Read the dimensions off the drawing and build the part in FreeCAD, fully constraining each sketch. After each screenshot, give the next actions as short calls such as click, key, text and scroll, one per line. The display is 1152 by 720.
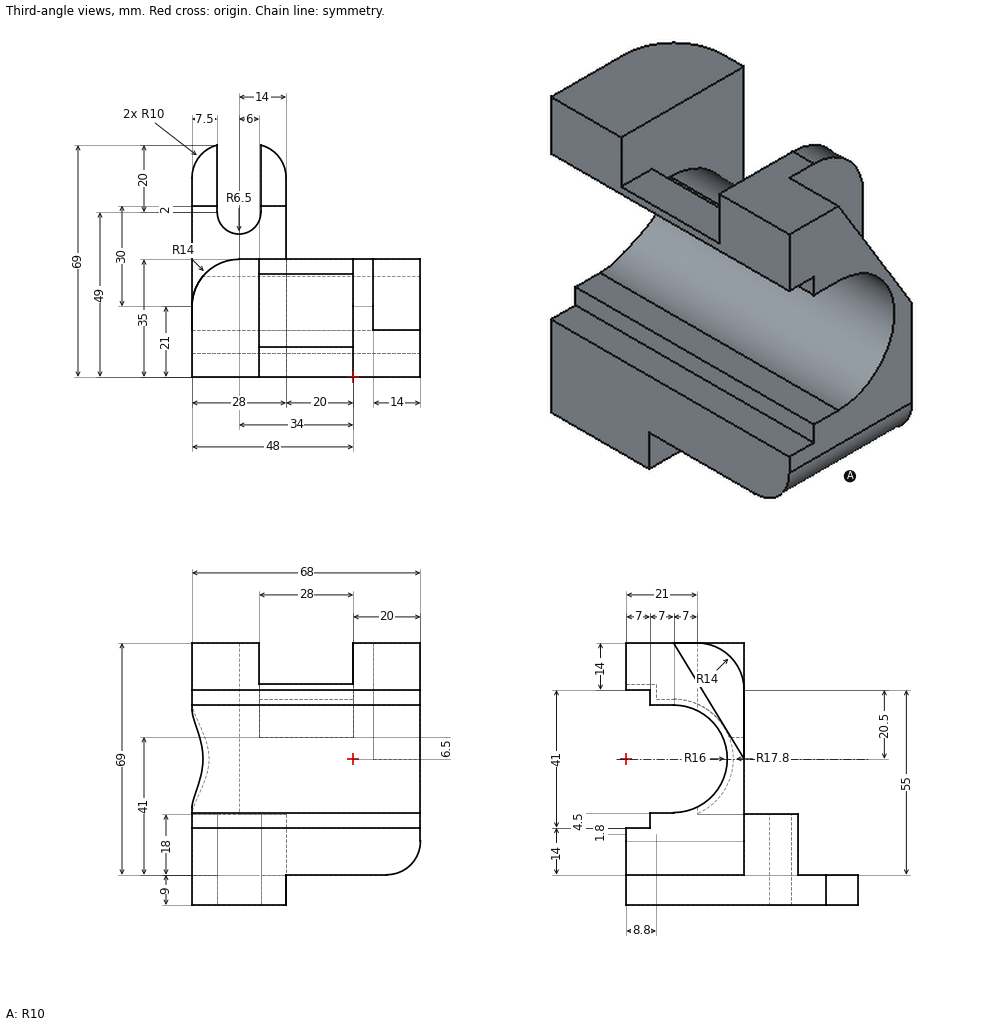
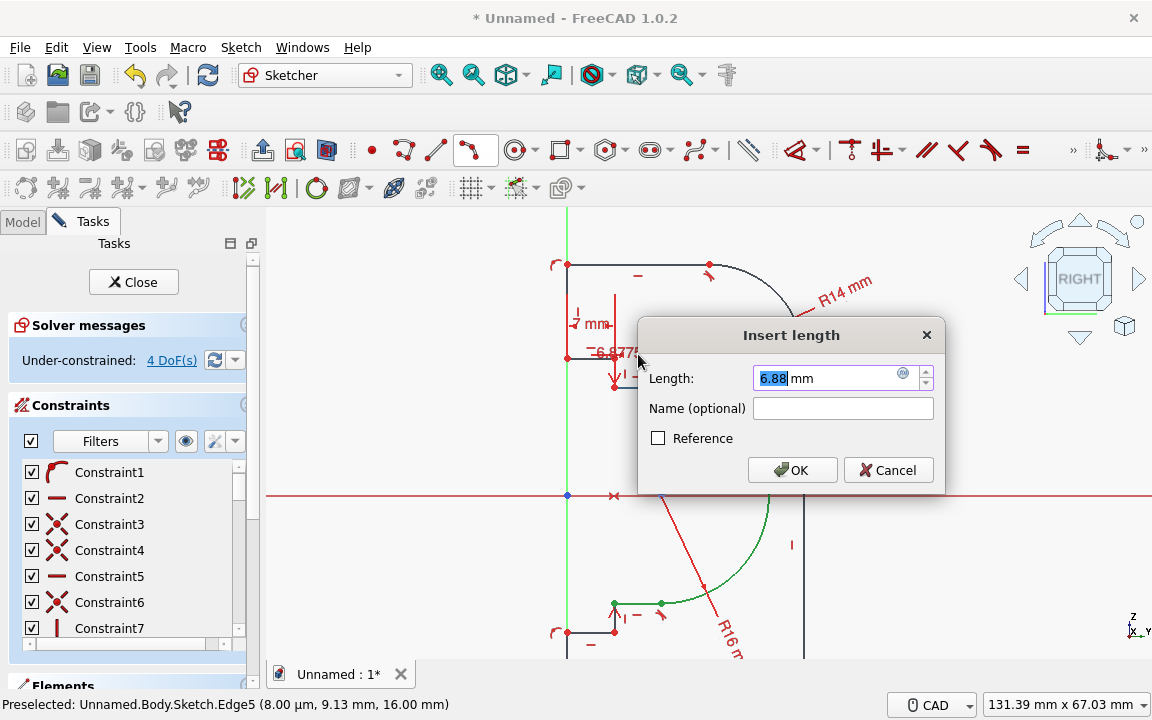
text(7)
key(Return)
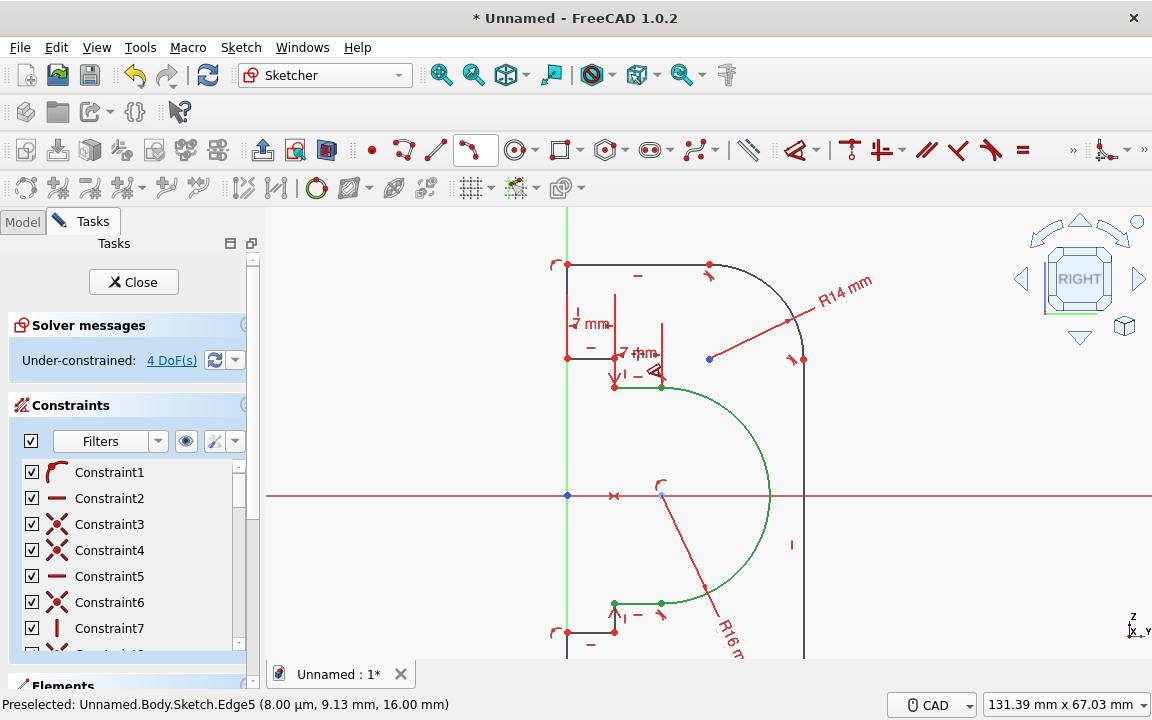
click(667, 265)
click(638, 299)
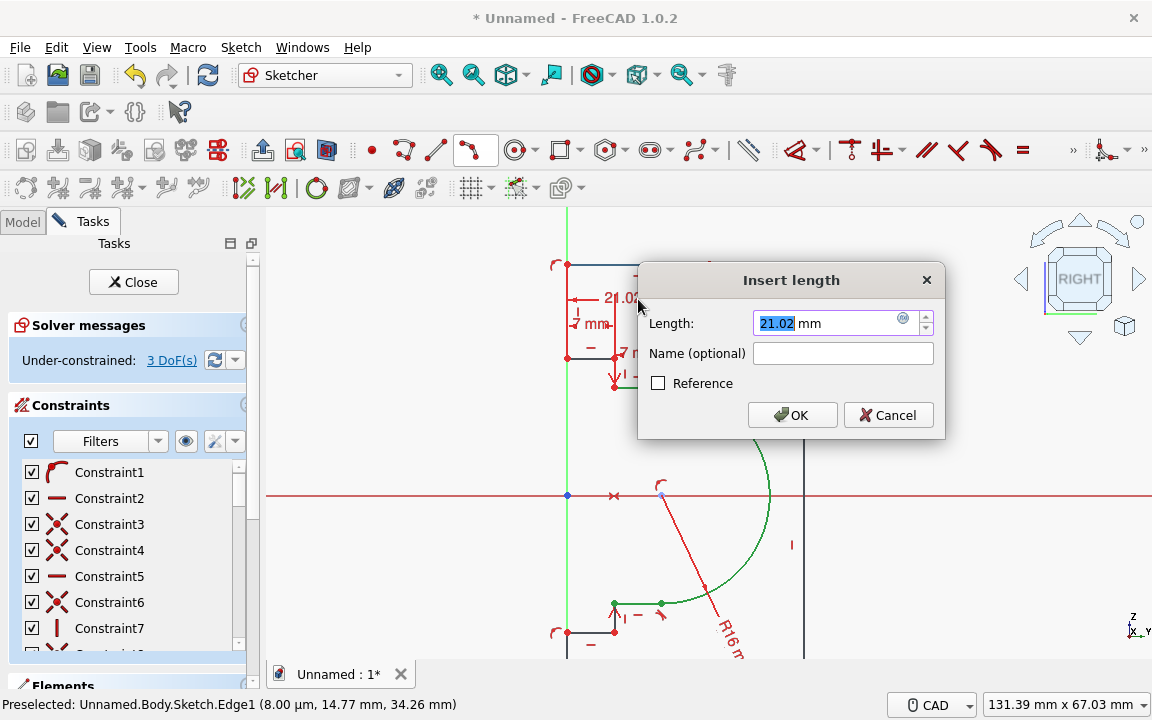
text(21)
key(Return)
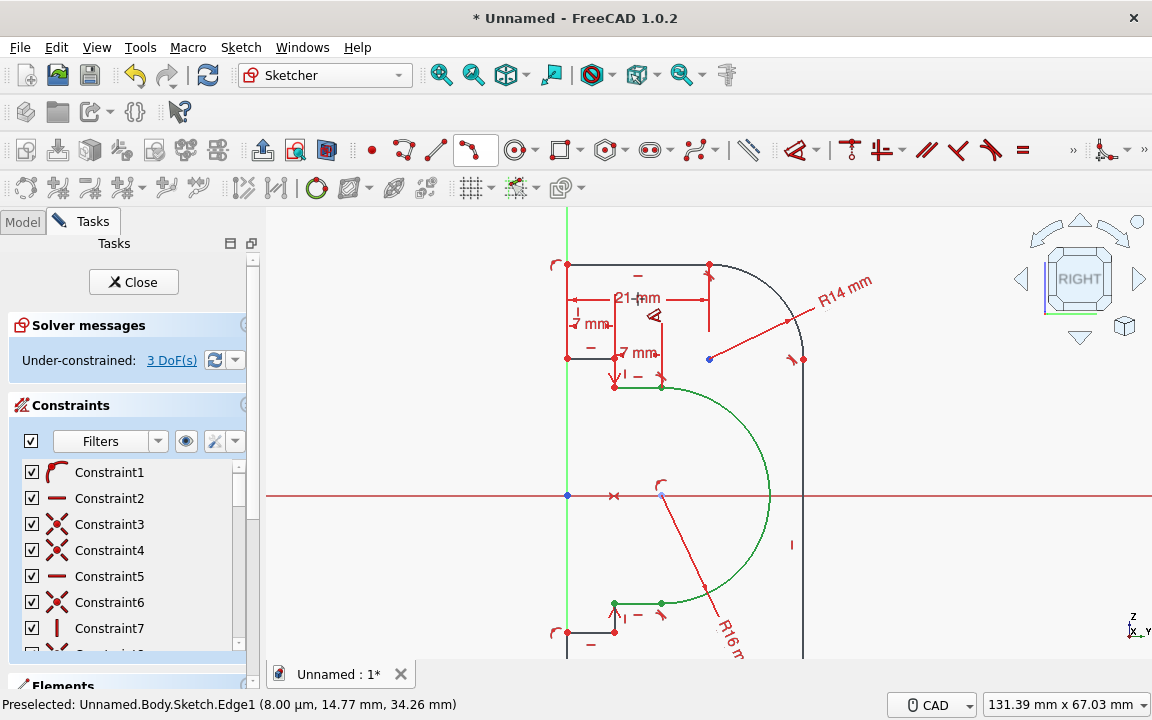
click(567, 293)
click(533, 290)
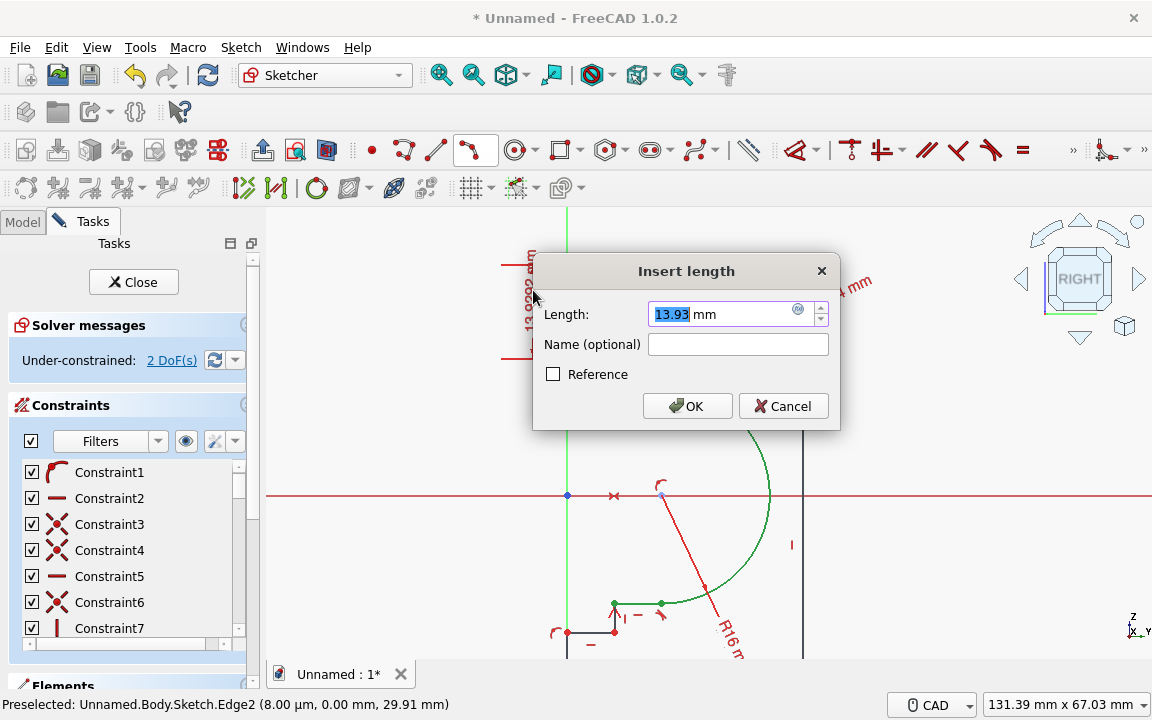
text(14)
key(Return)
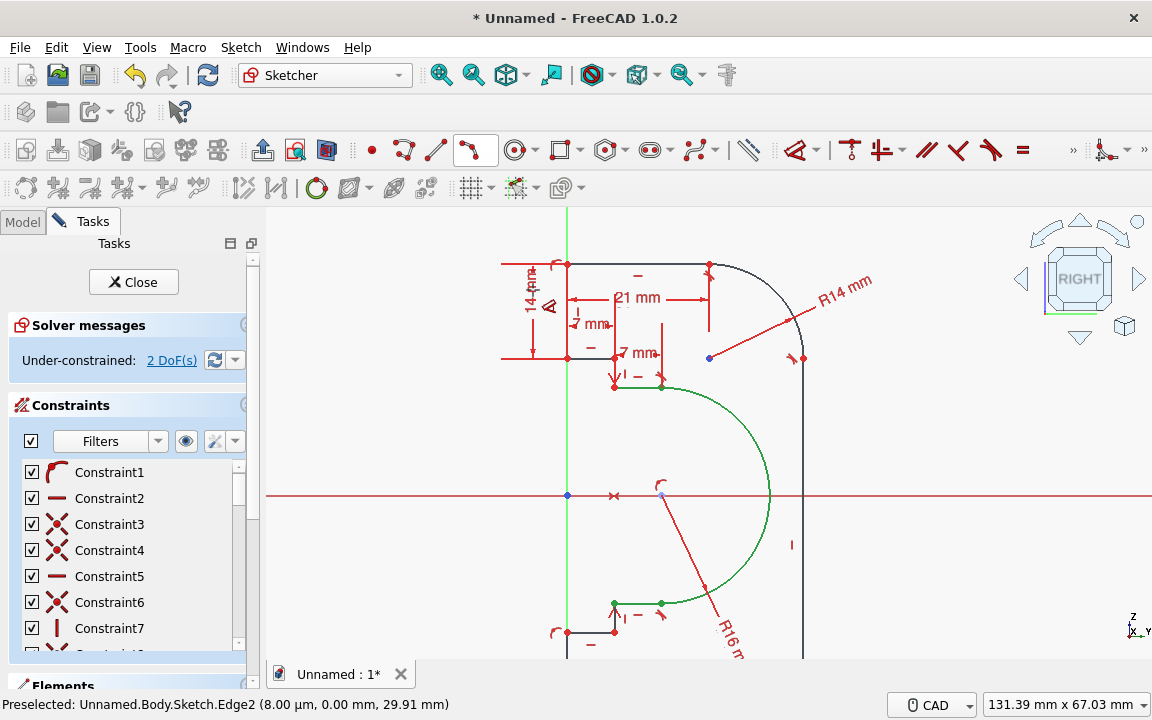
scroll(586, 357, down, 3)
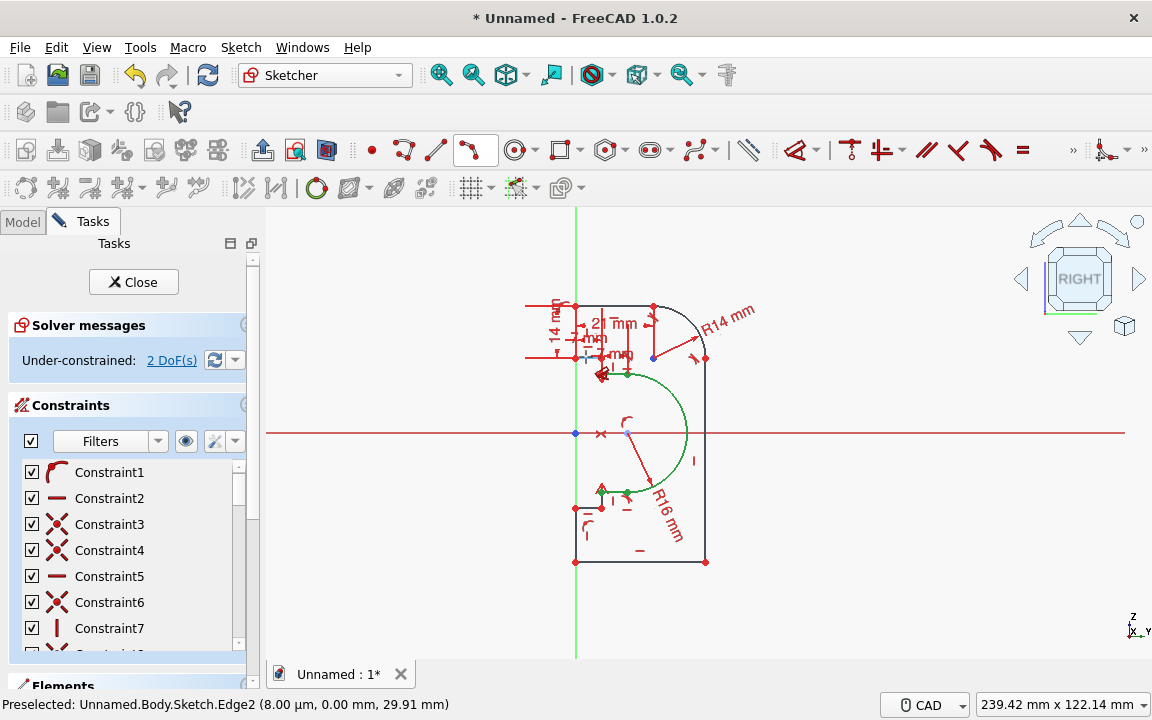
click(576, 525)
click(542, 535)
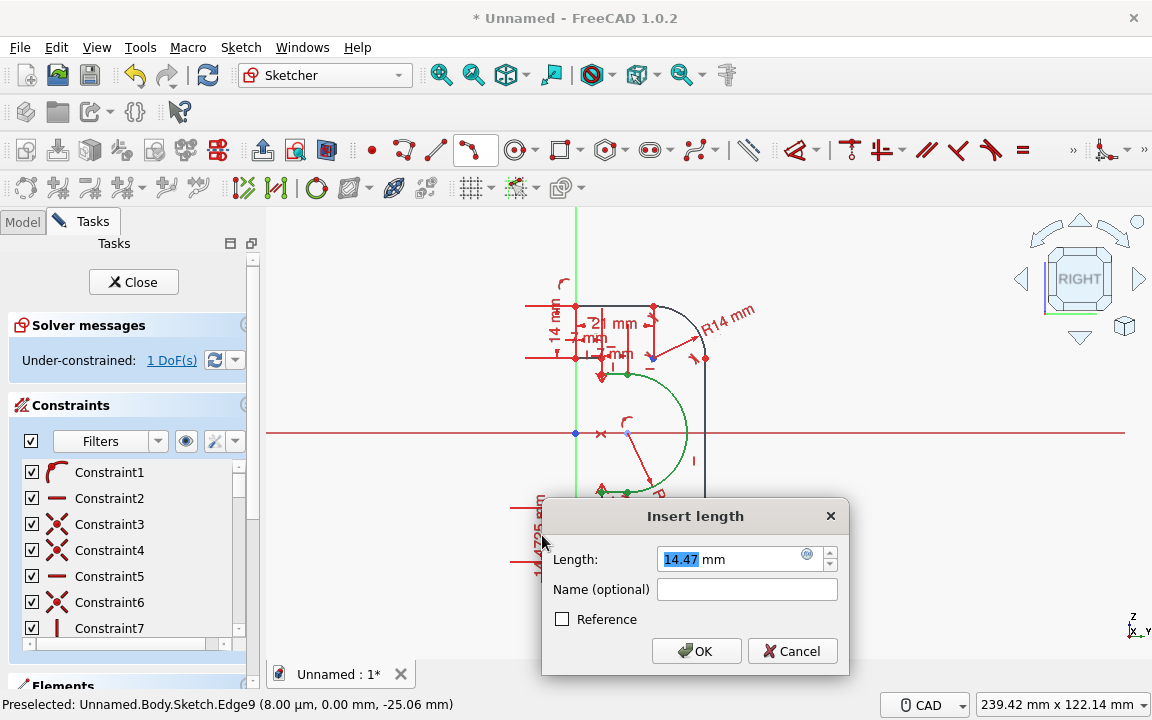
text(14)
key(Return)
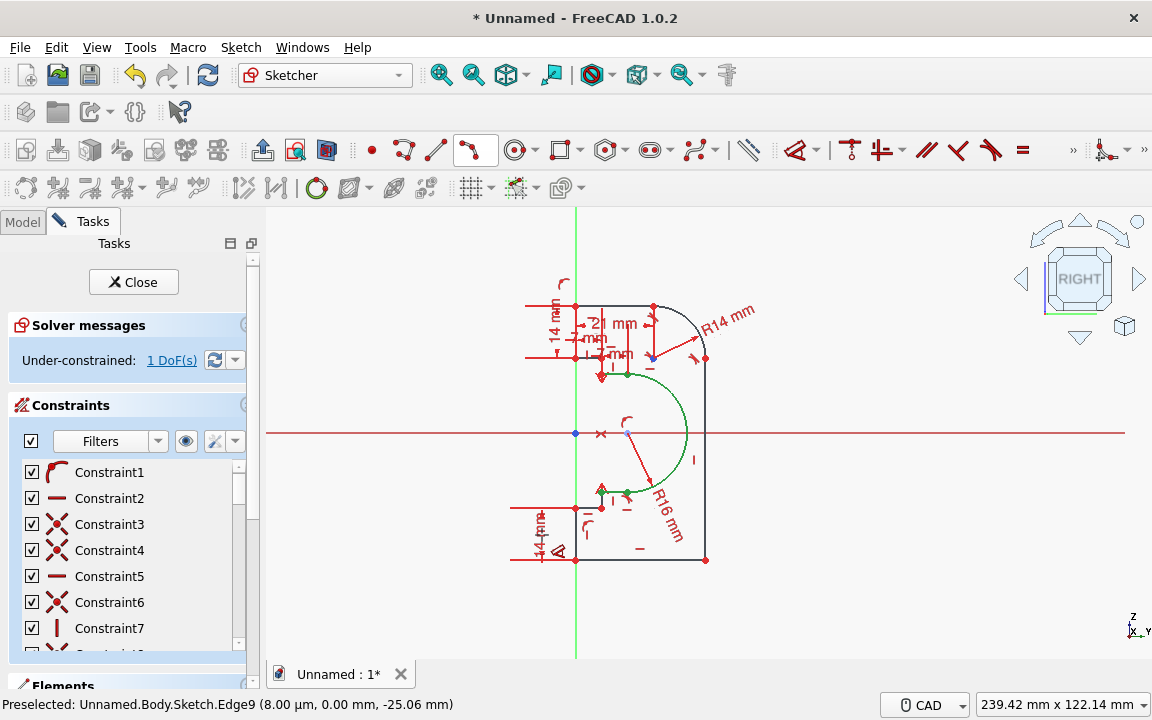
click(705, 500)
click(739, 459)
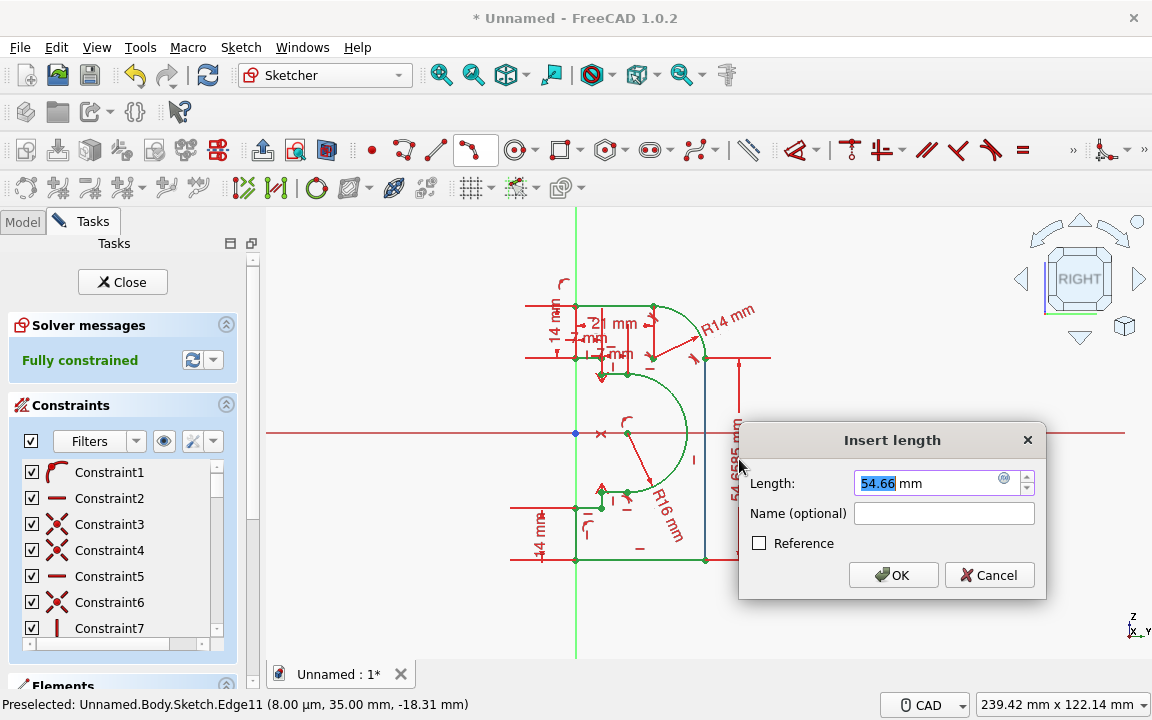
text(55)
key(Return)
key(Escape)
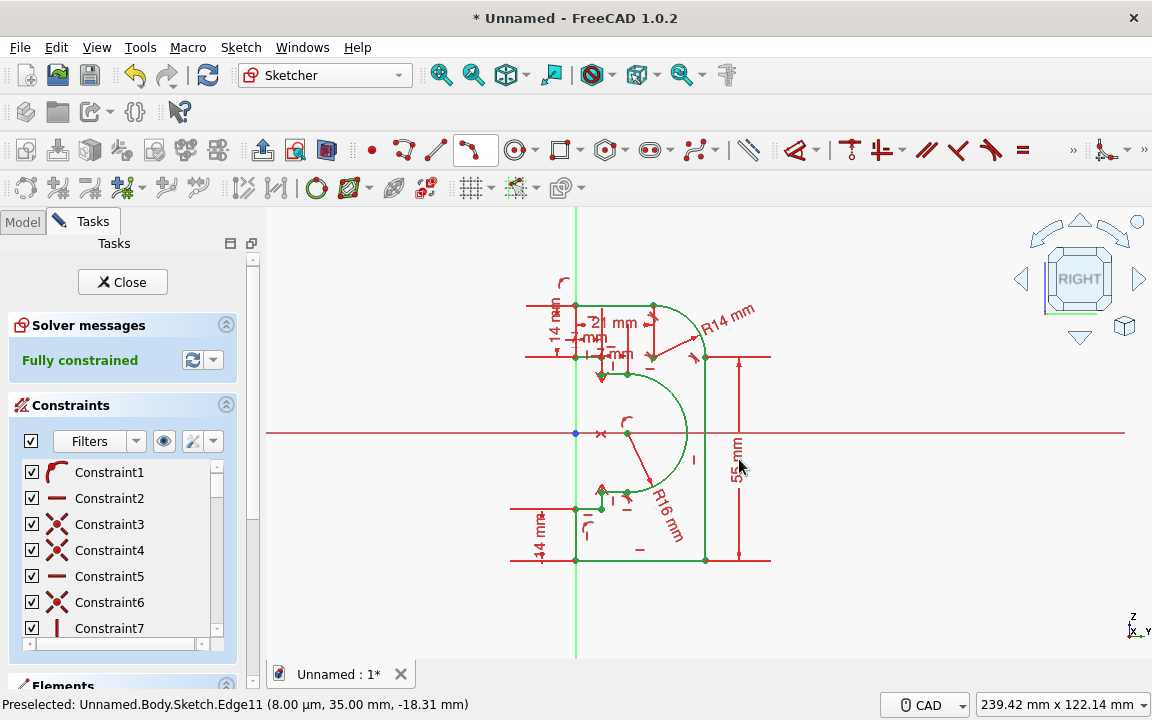
click(123, 282)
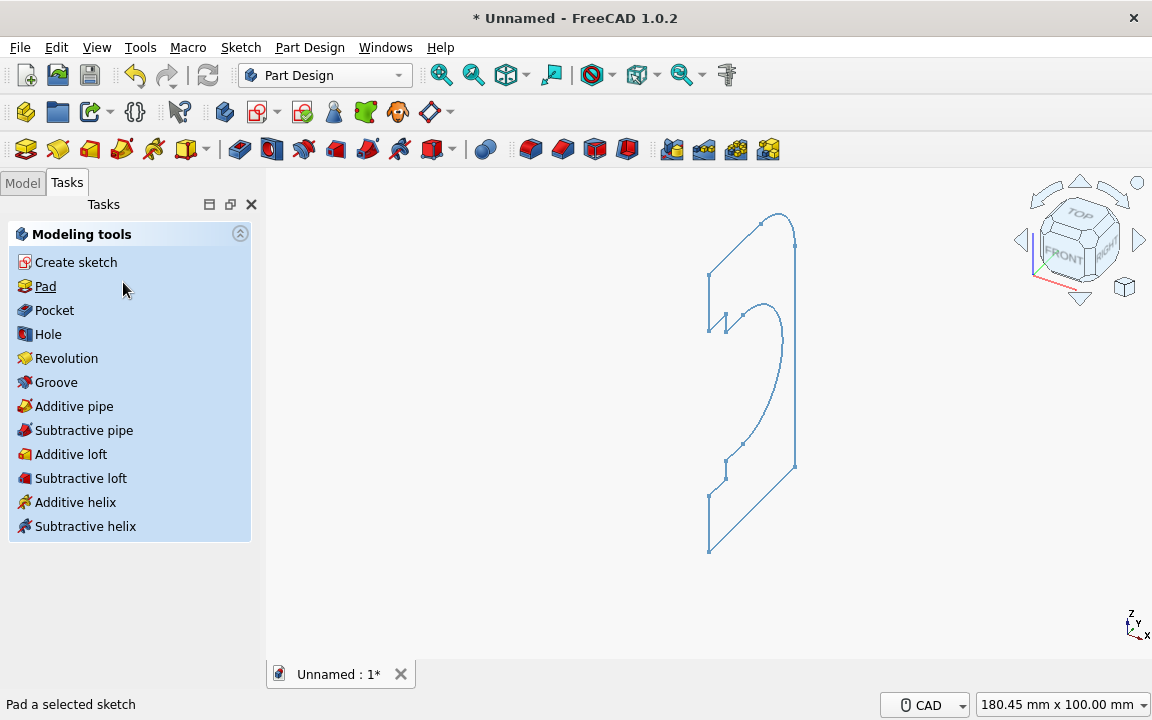
click(26, 150)